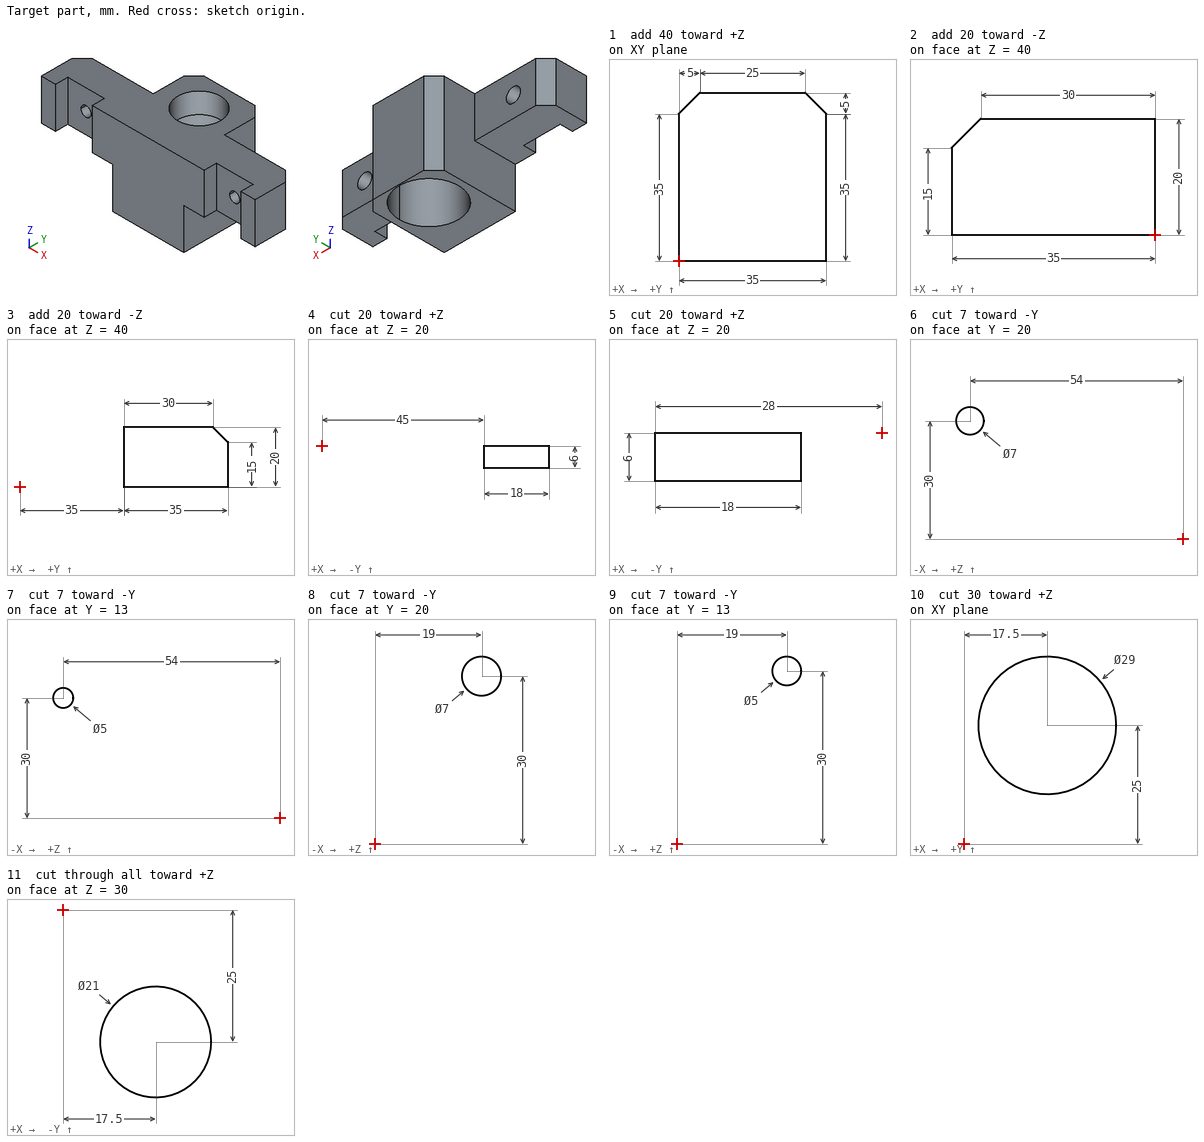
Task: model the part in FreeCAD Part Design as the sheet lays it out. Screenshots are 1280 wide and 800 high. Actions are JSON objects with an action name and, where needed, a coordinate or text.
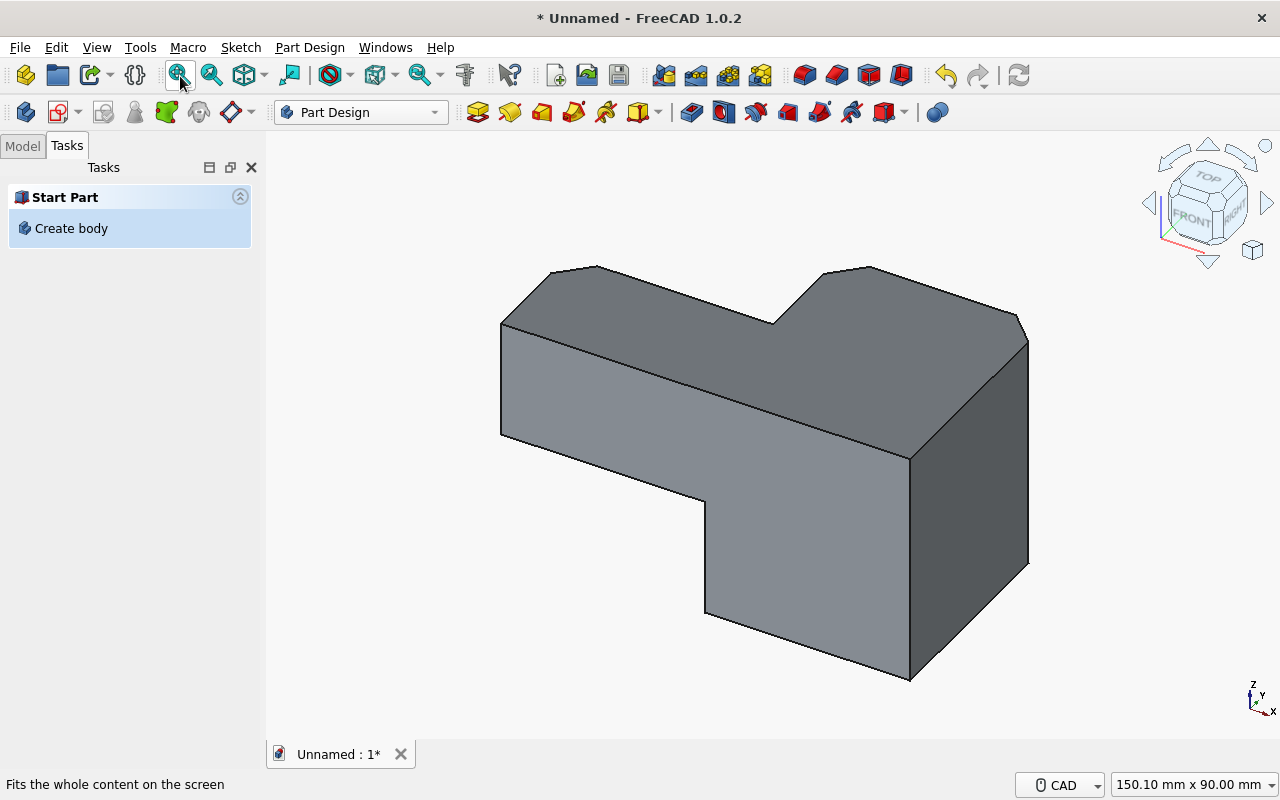
{"action": "left_click", "coordinate": [890, 362]}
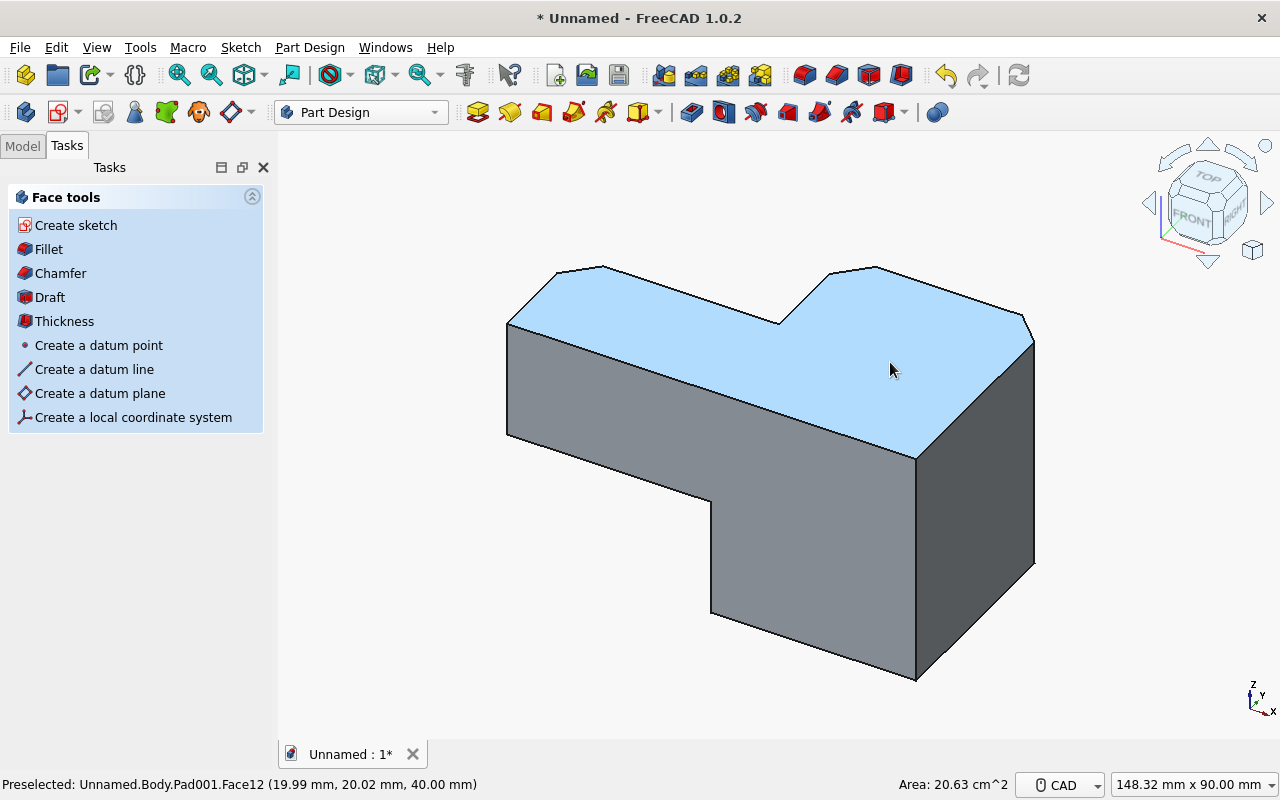
{"action": "left_click", "coordinate": [58, 112]}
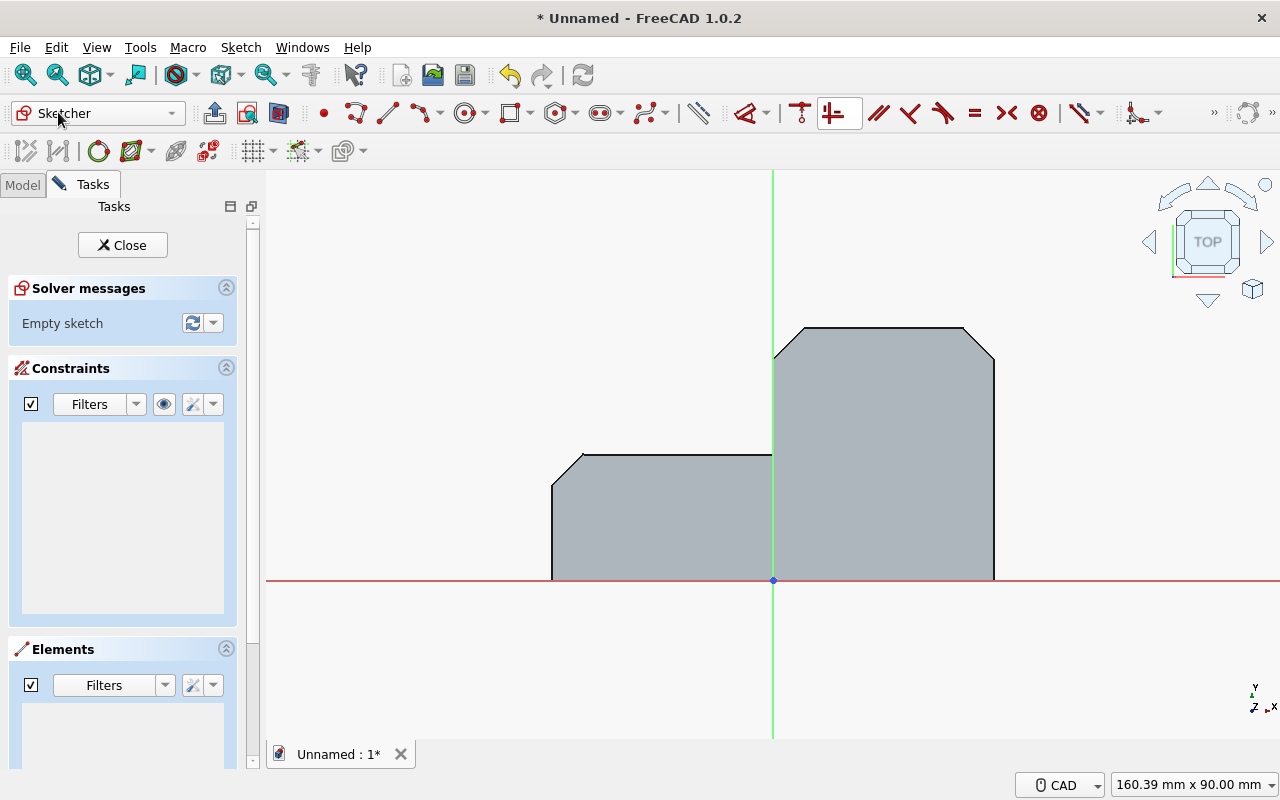
{"action": "scroll", "coordinate": [294, 198], "scroll_direction": "down", "scroll_amount": 1}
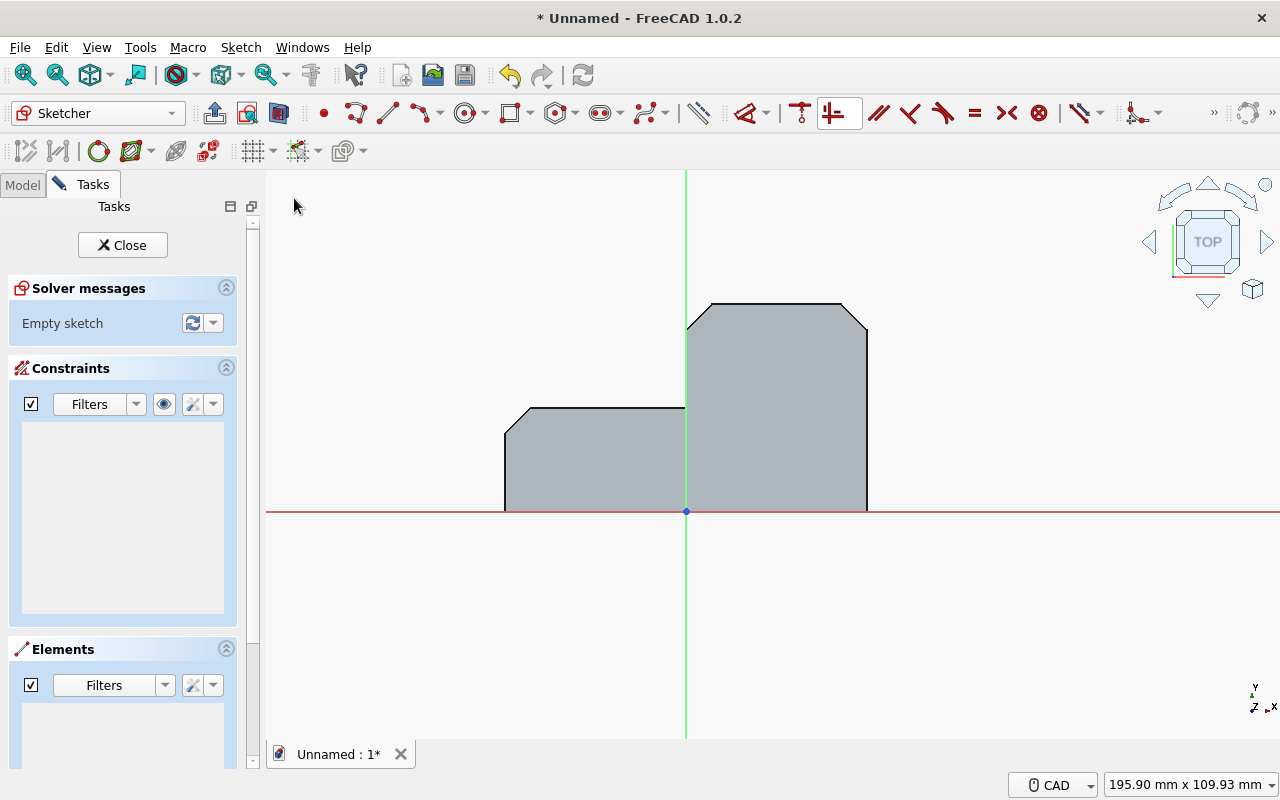
{"action": "scroll", "coordinate": [1115, 471], "scroll_direction": "up", "scroll_amount": 2}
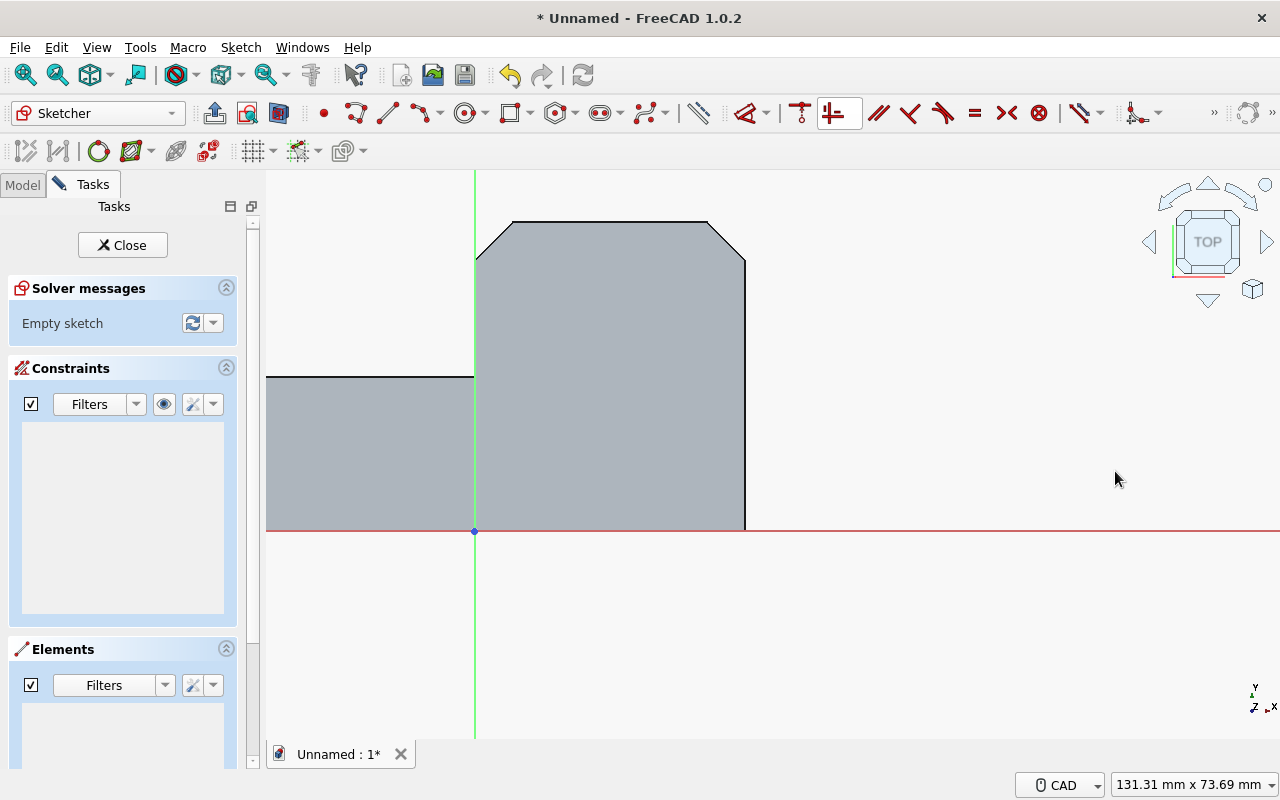
{"action": "left_click", "coordinate": [356, 114]}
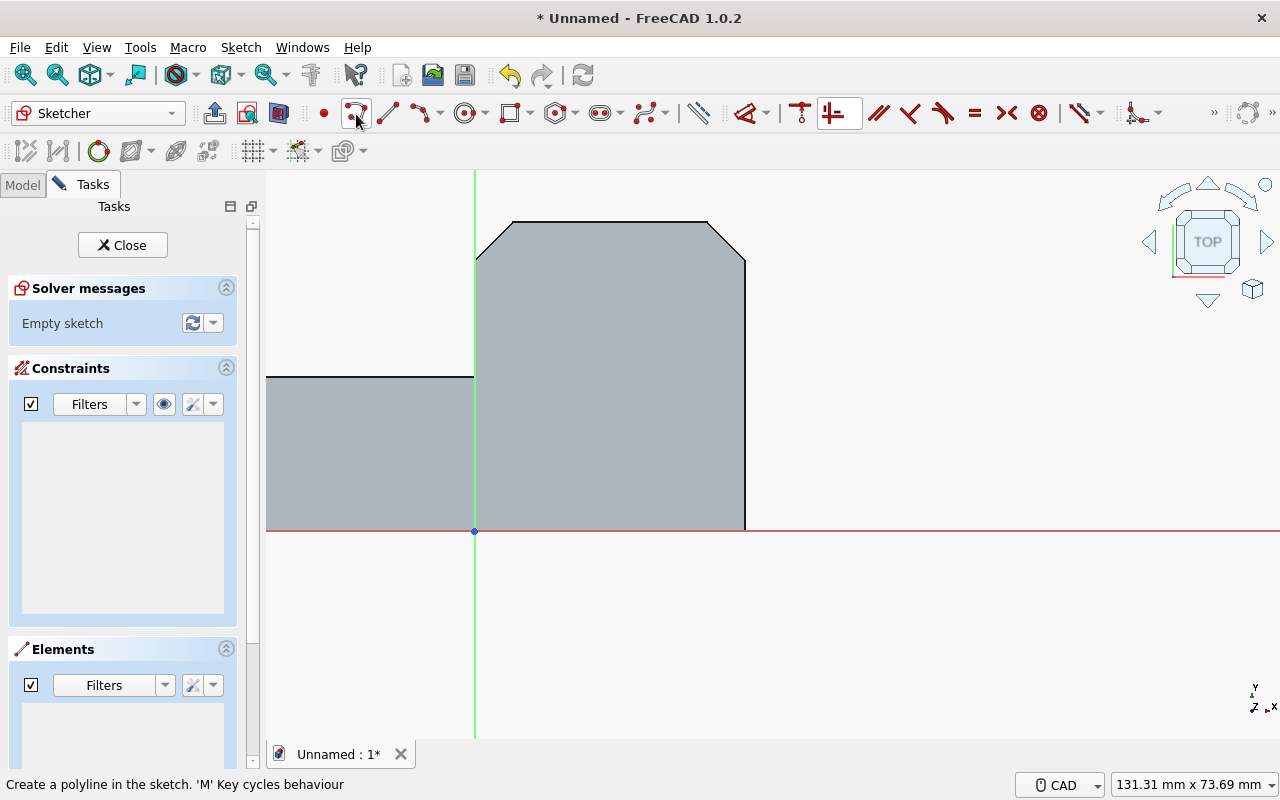
{"action": "left_click", "coordinate": [745, 531]}
{"action": "left_click", "coordinate": [1015, 522]}
{"action": "left_click", "coordinate": [1015, 415]}
{"action": "left_click", "coordinate": [977, 377]}
{"action": "left_click", "coordinate": [745, 377]}
{"action": "left_click", "coordinate": [745, 531]}
{"action": "key", "text": "Escape"}
{"action": "key", "text": "Escape"}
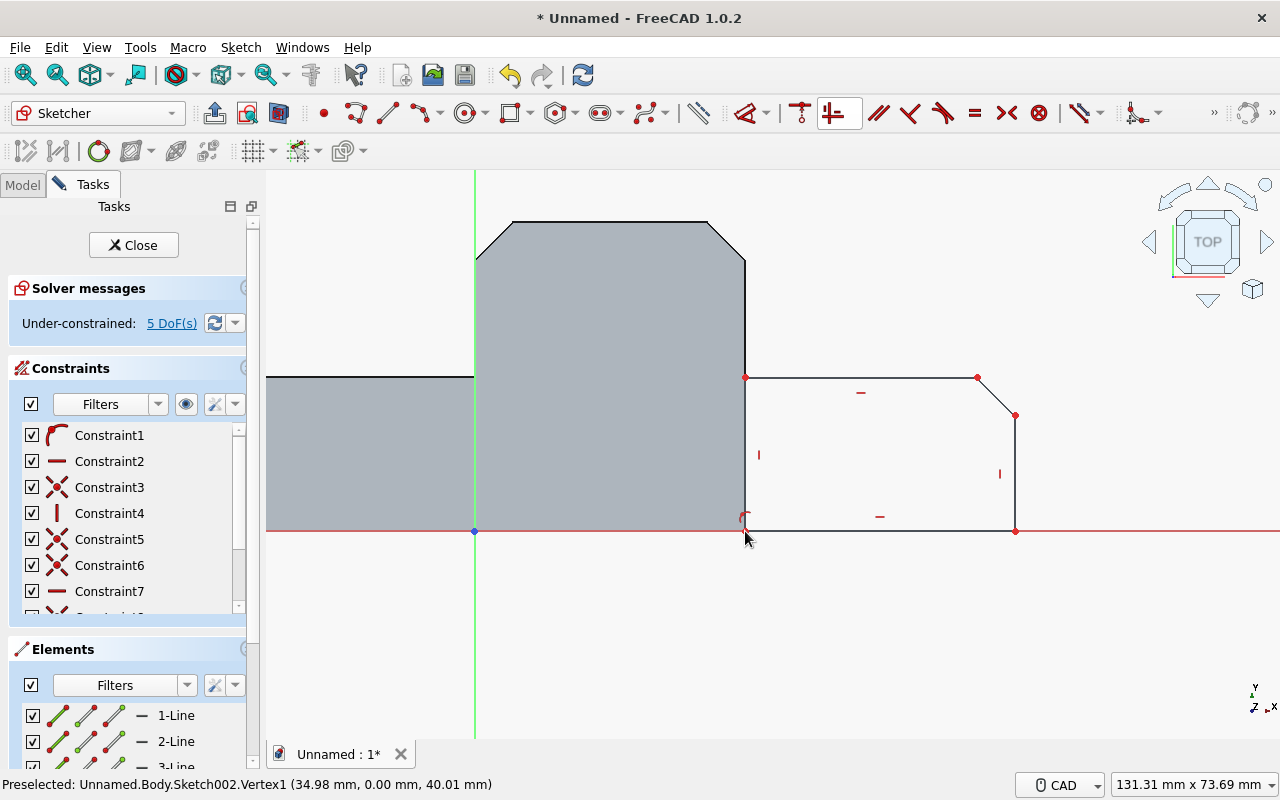
{"action": "left_click", "coordinate": [746, 114]}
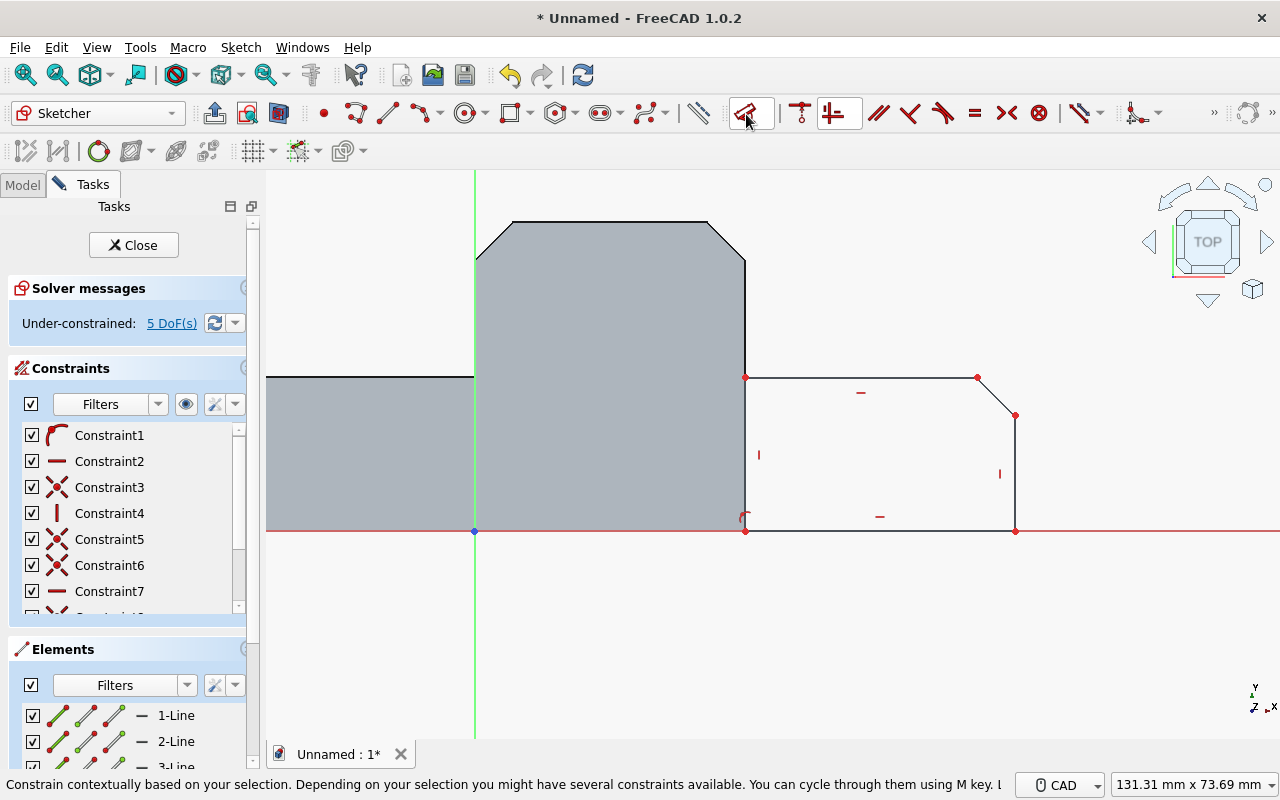
{"action": "left_click", "coordinate": [826, 531]}
{"action": "left_click", "coordinate": [880, 565]}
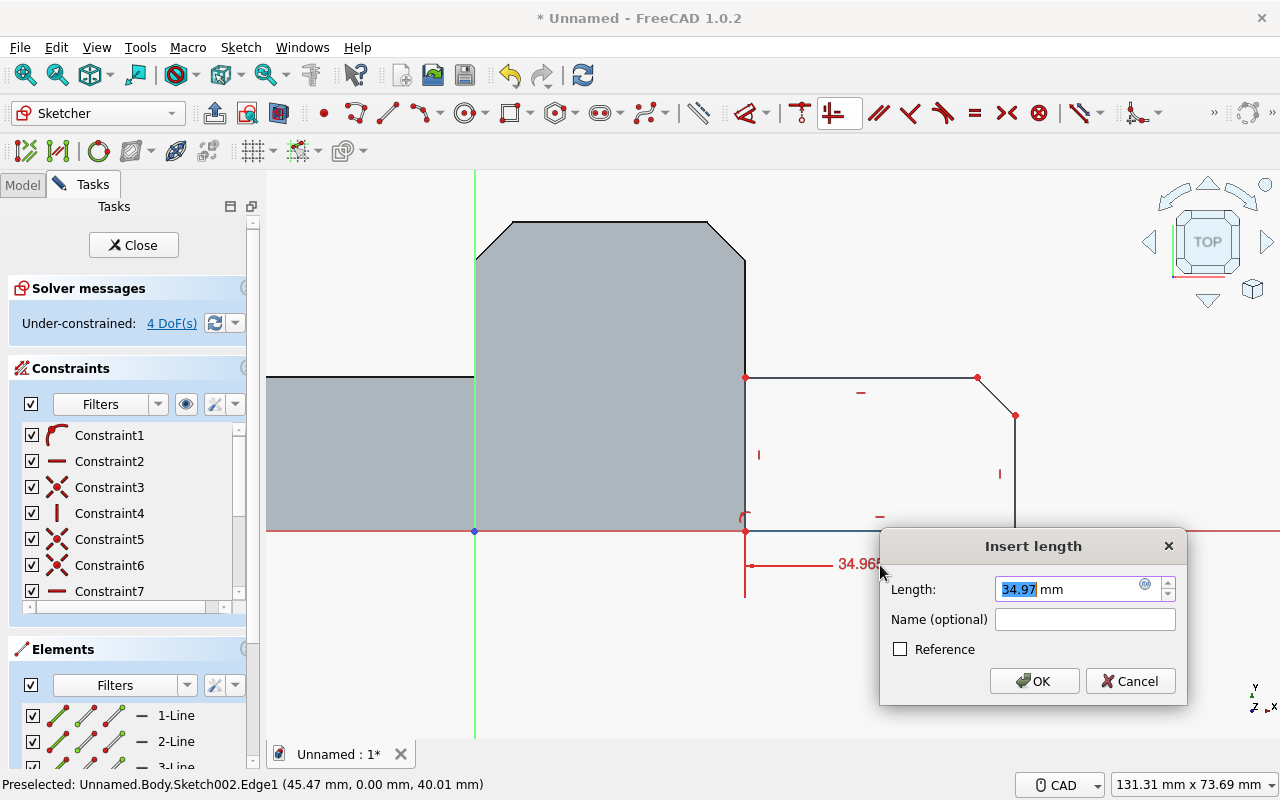
{"action": "type", "text": "35"}
{"action": "key", "text": "Return"}